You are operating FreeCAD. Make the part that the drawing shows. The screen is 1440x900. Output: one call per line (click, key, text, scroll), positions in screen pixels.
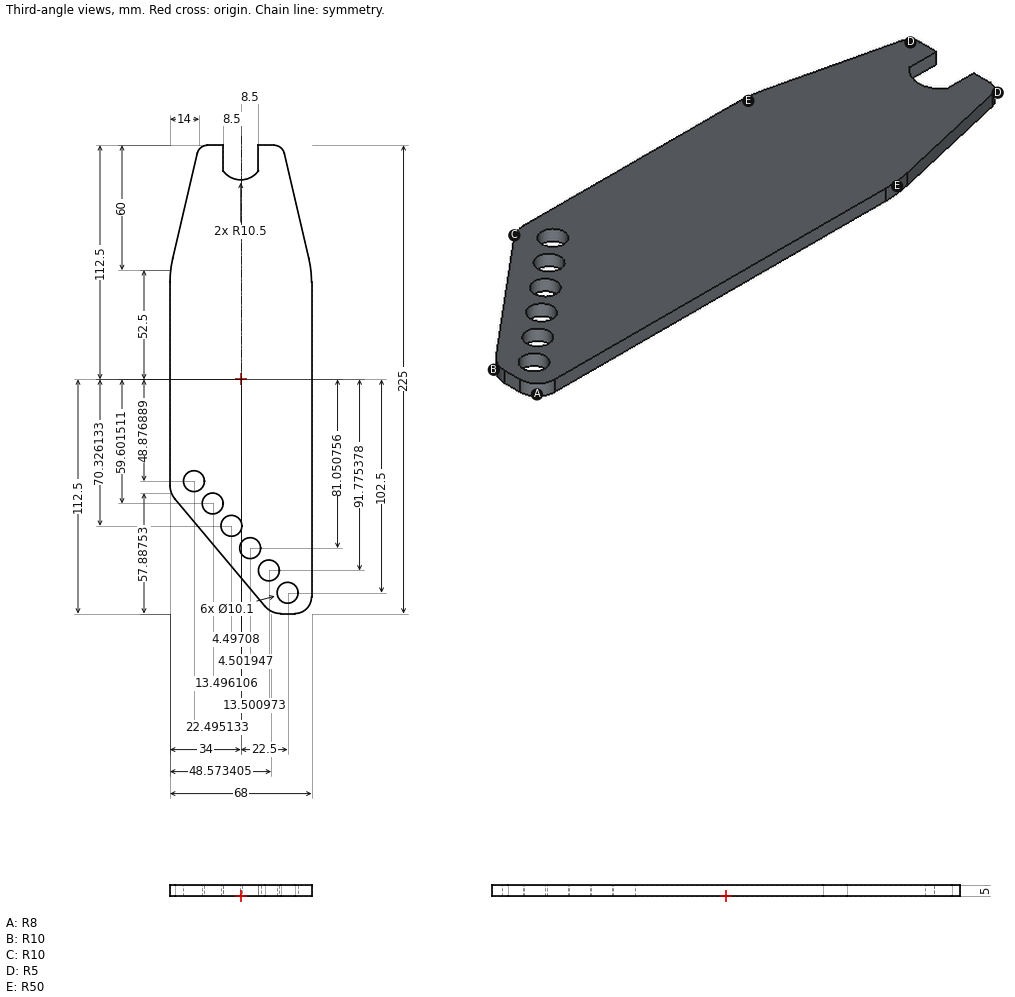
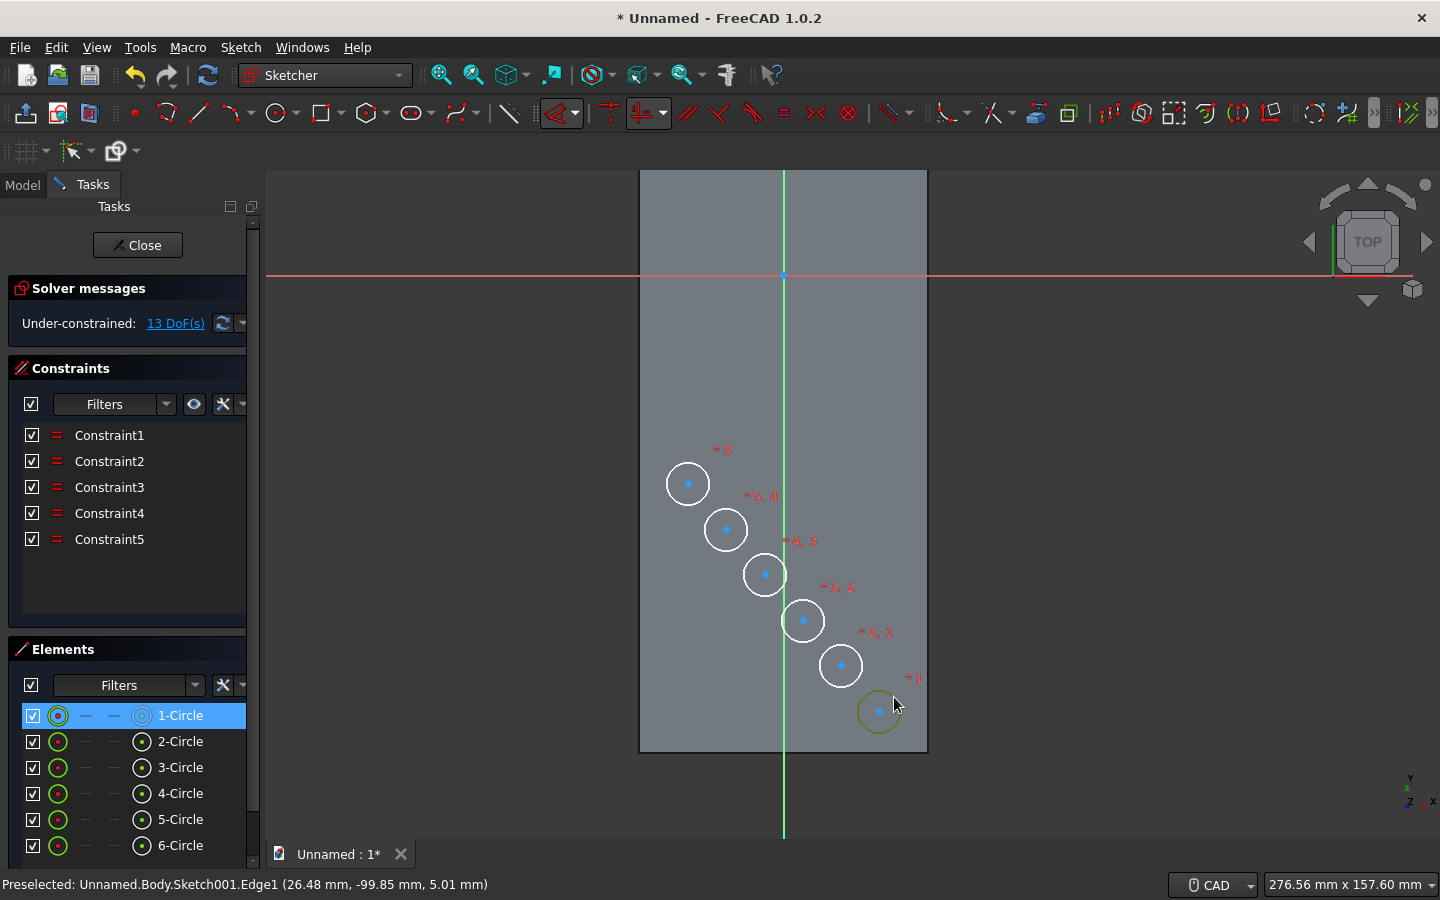
click(578, 114)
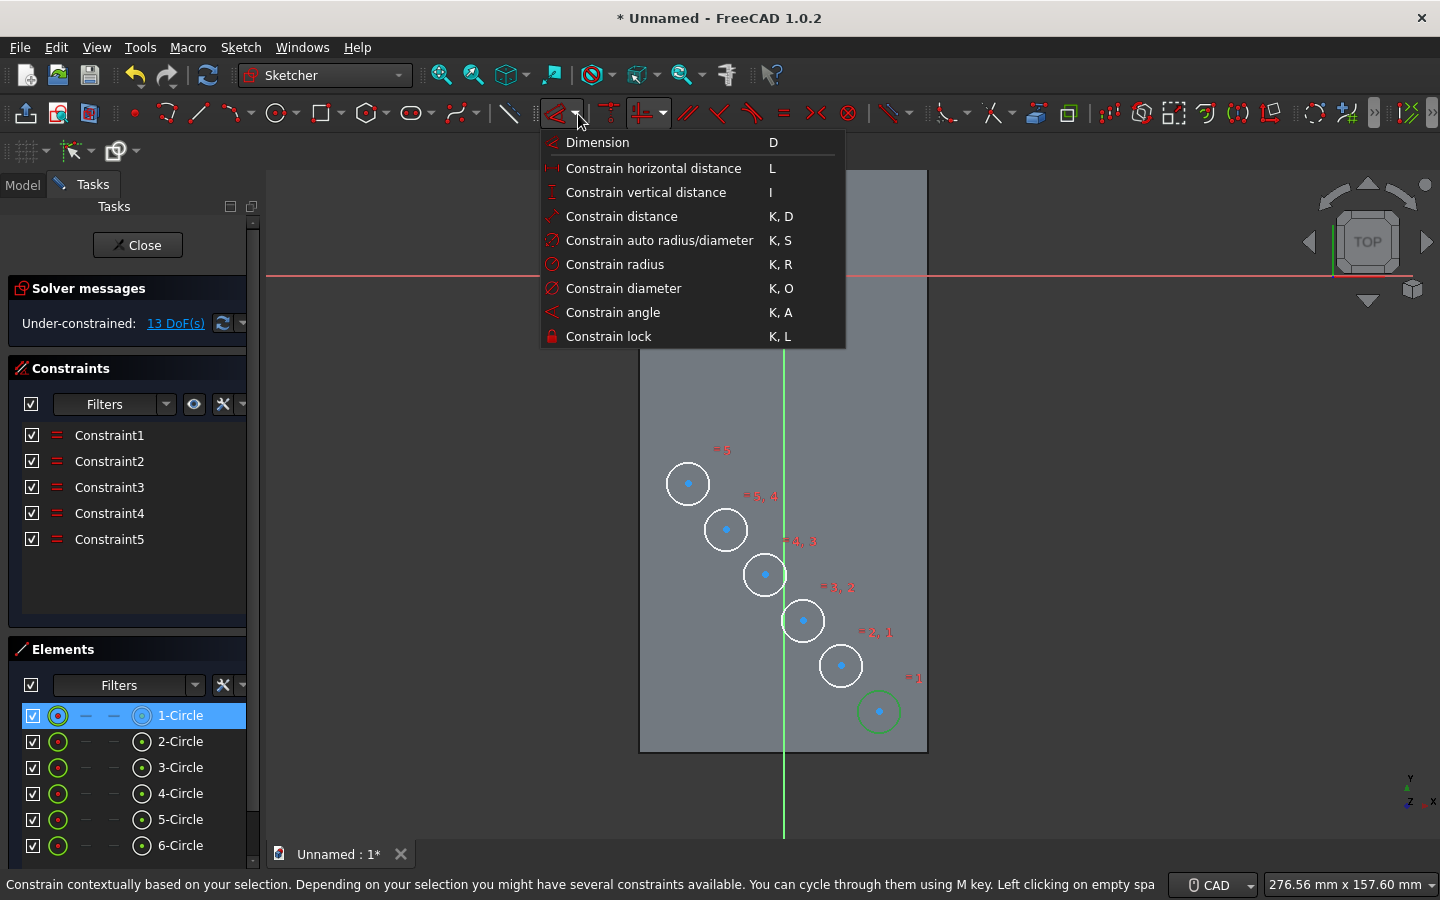
click(693, 288)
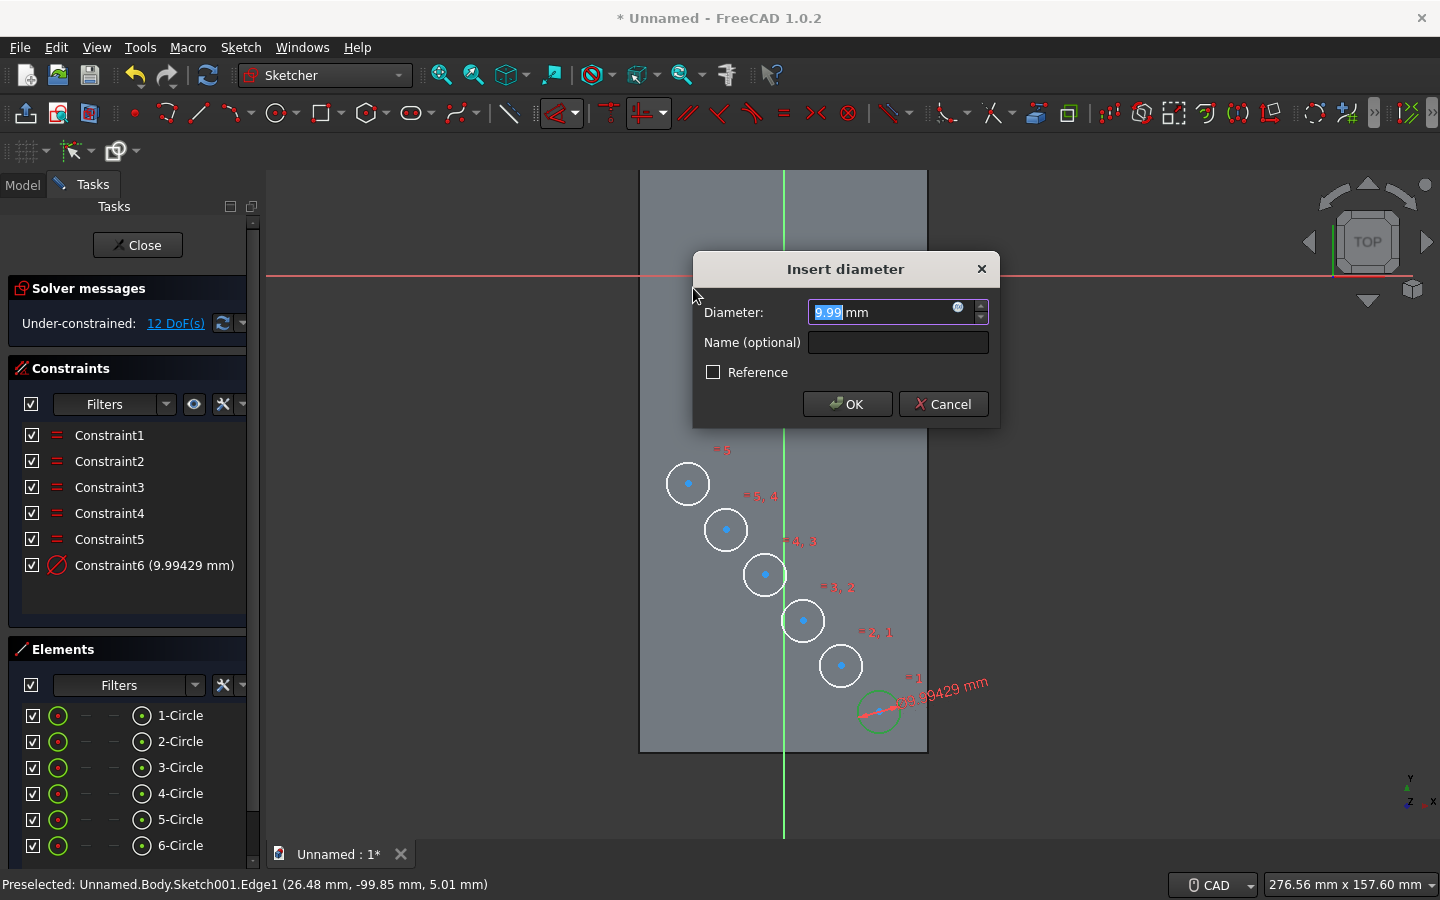
text(10.1)
key(Return)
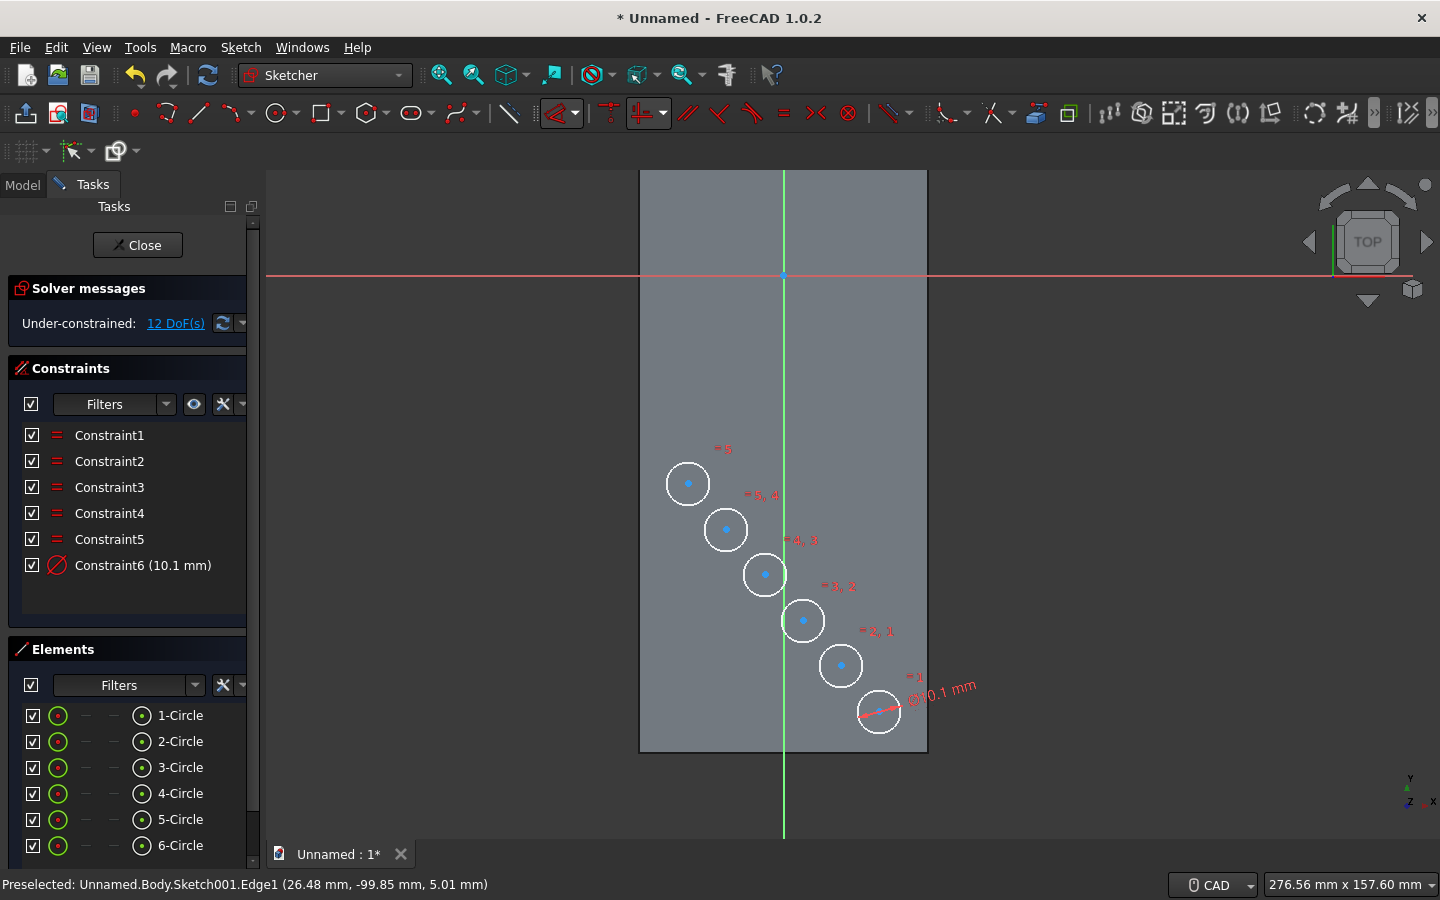
click(879, 712)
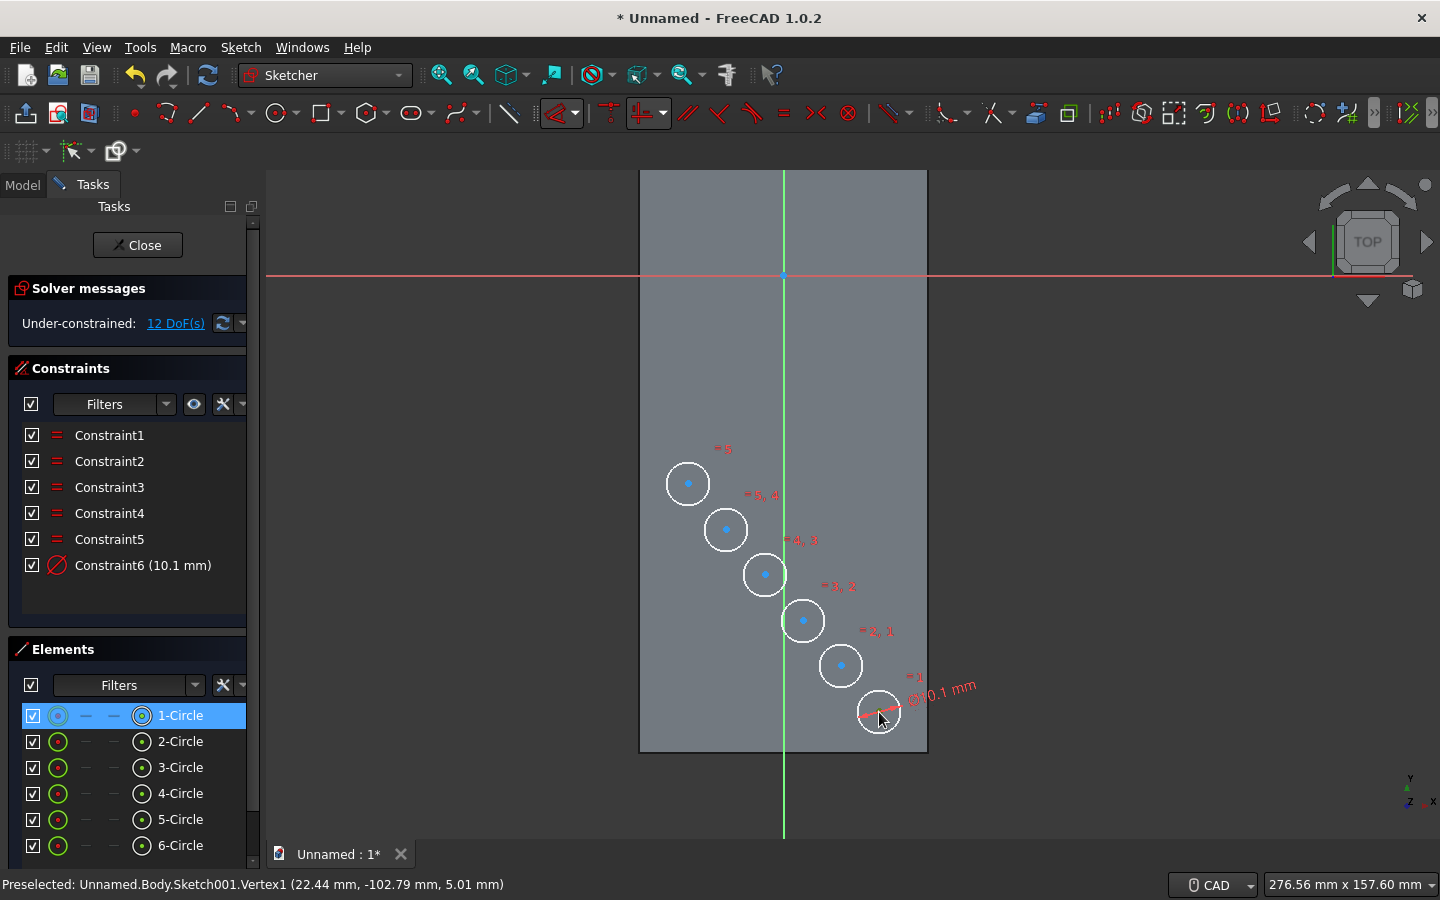
click(578, 114)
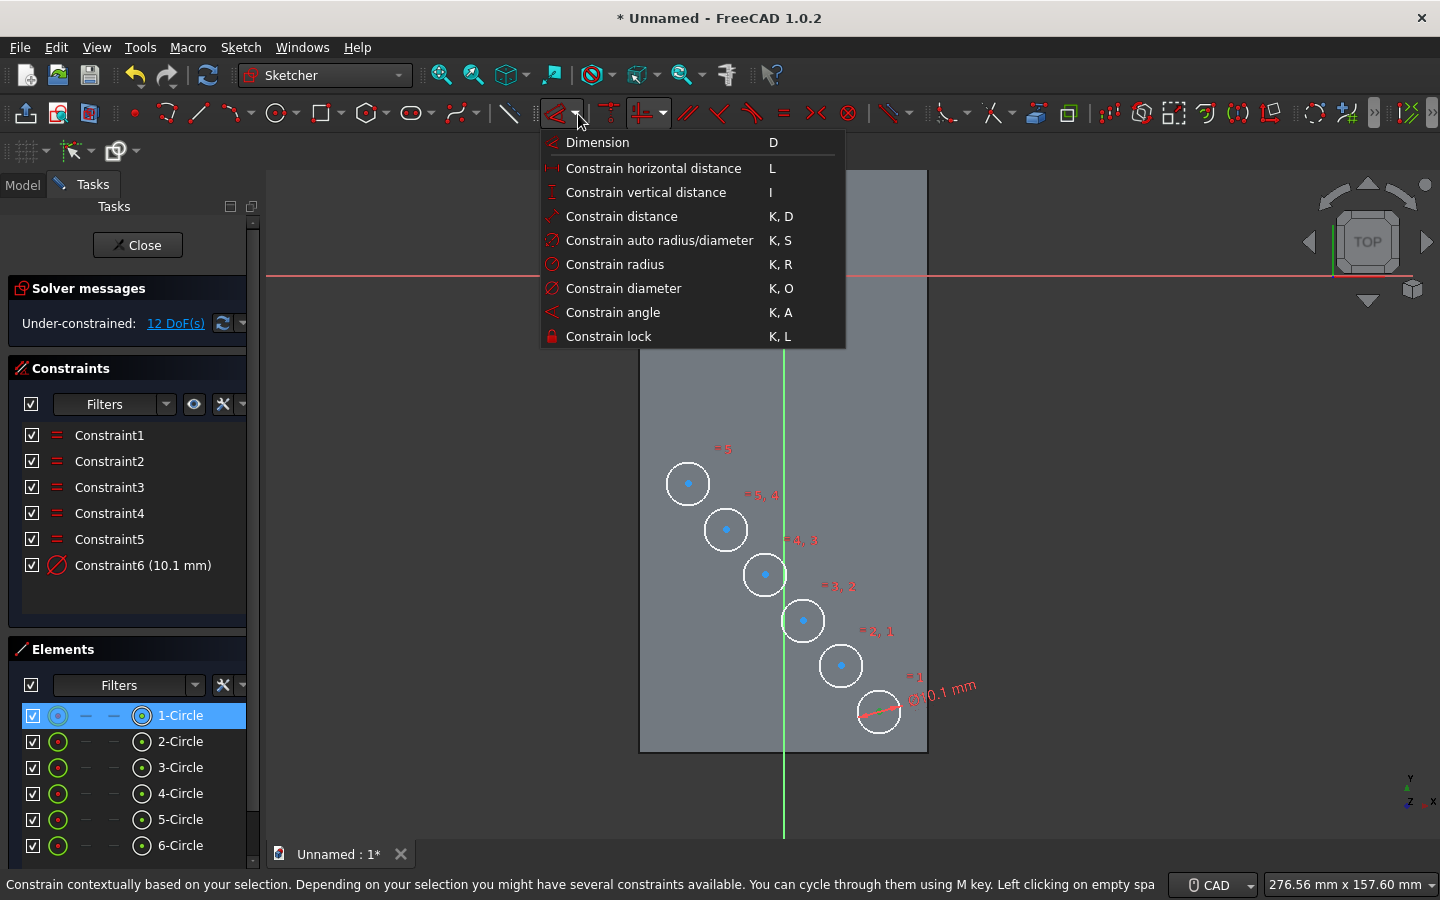
click(693, 168)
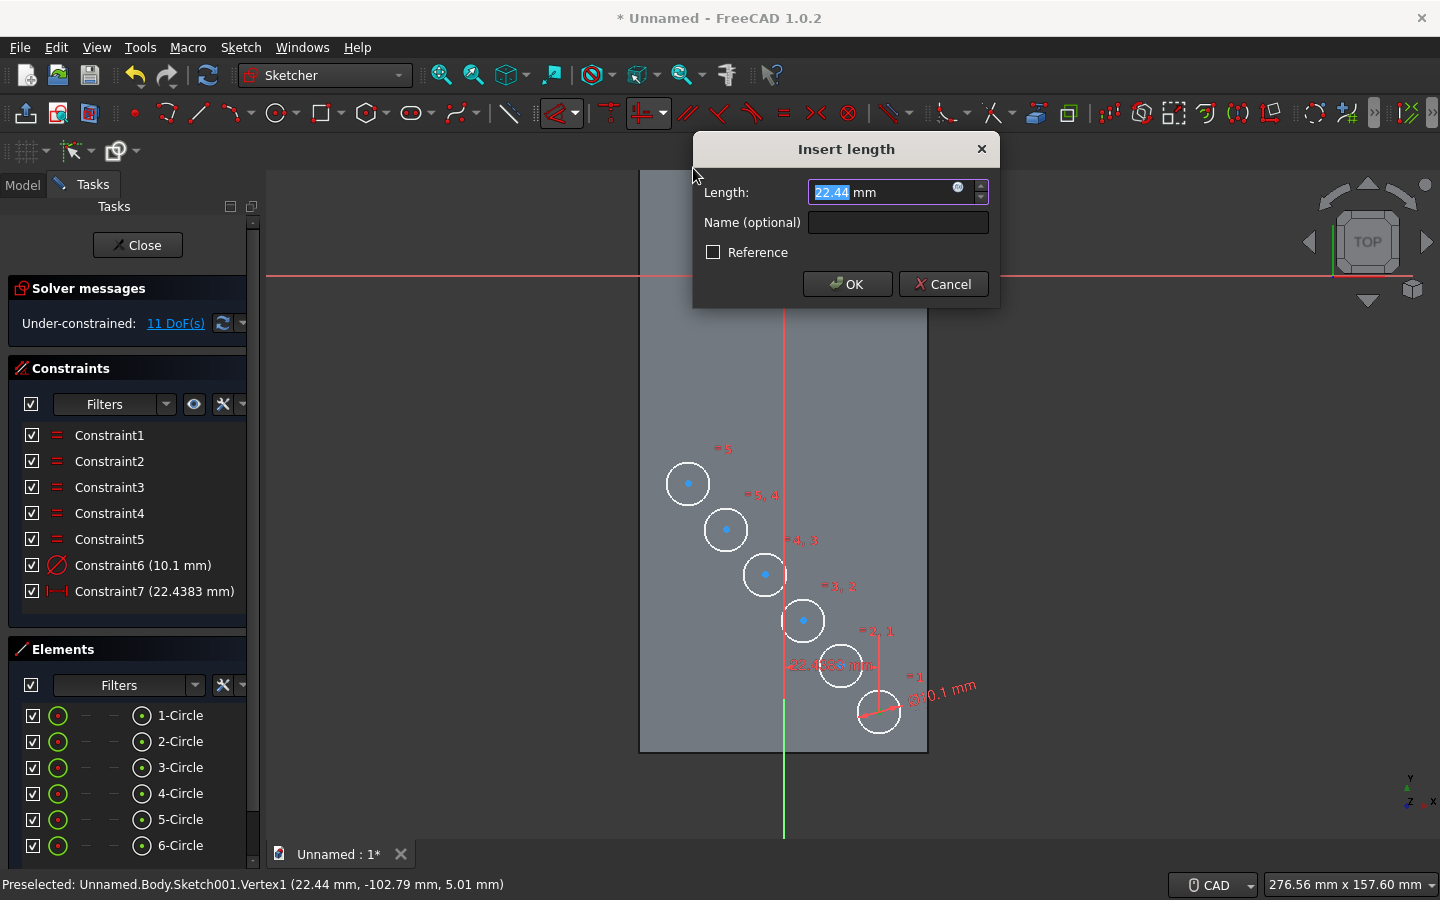
text(22.5)
key(Return)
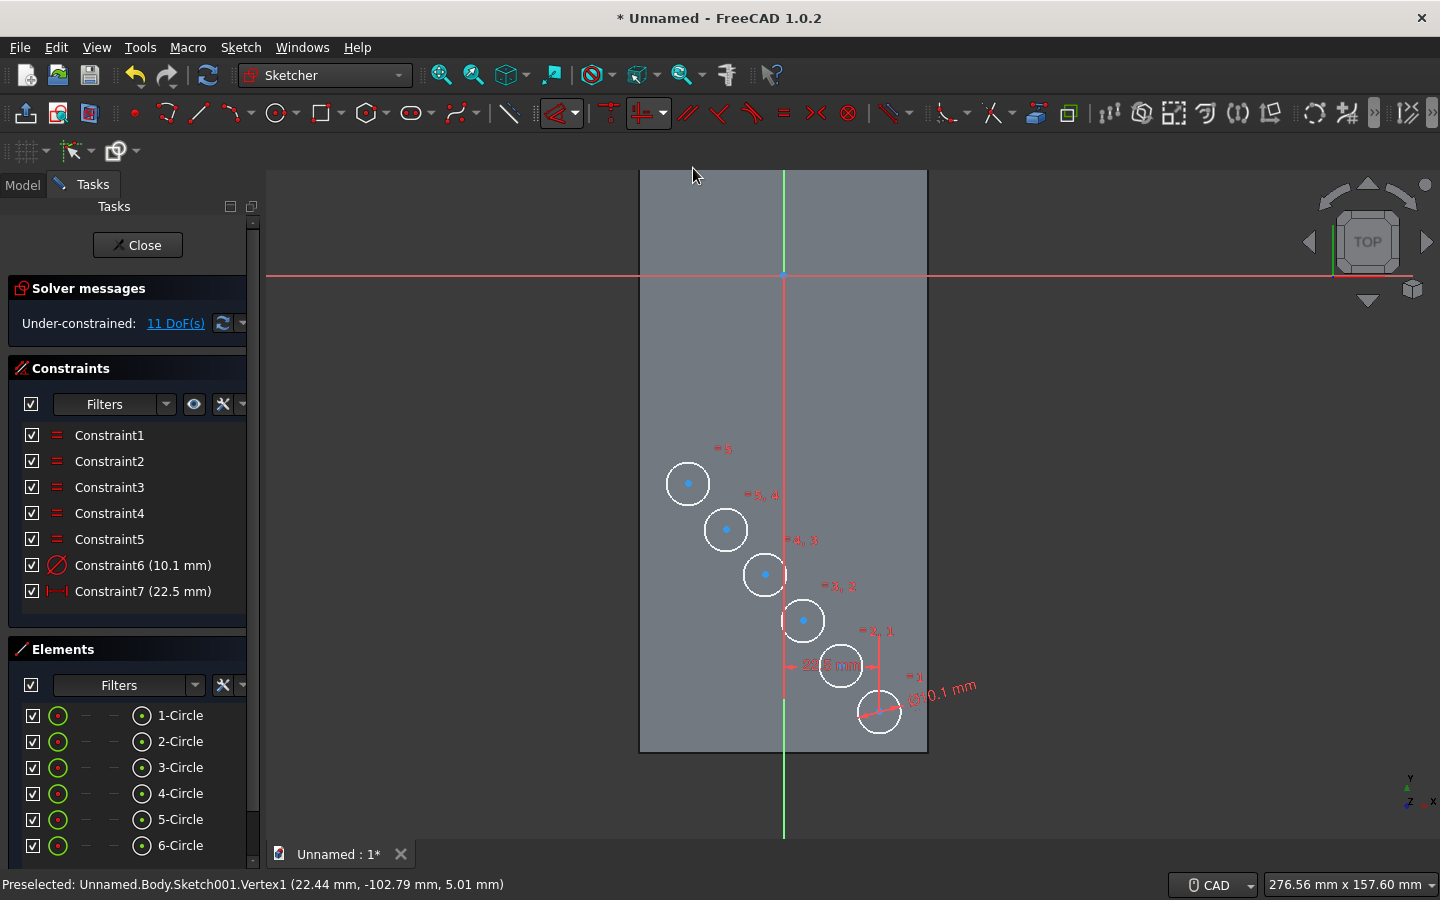
click(879, 712)